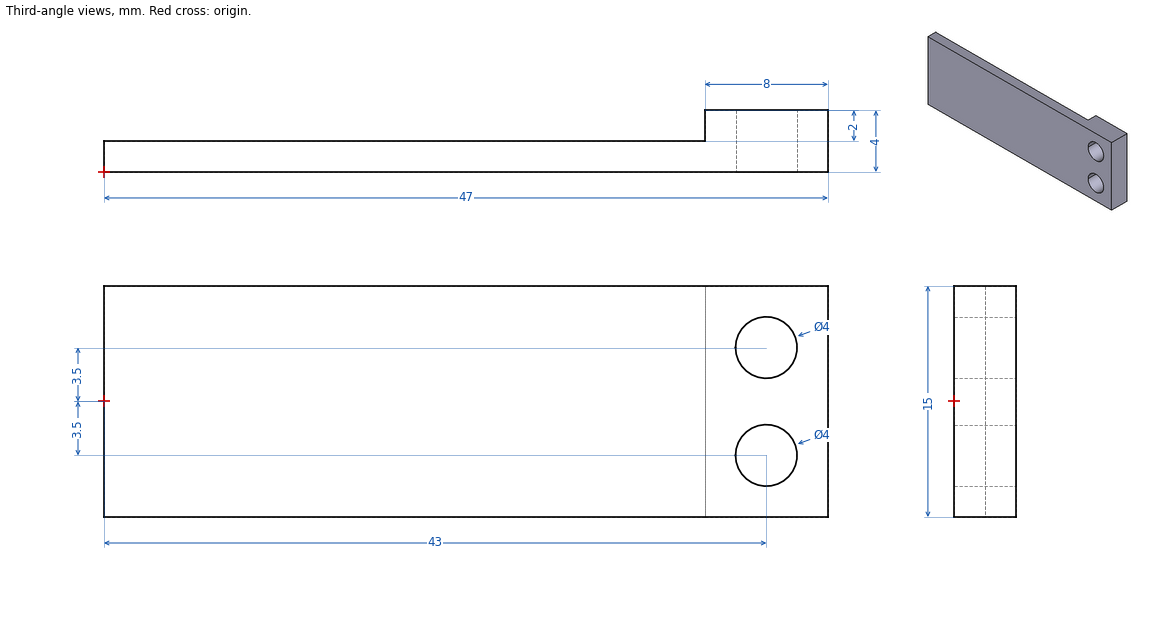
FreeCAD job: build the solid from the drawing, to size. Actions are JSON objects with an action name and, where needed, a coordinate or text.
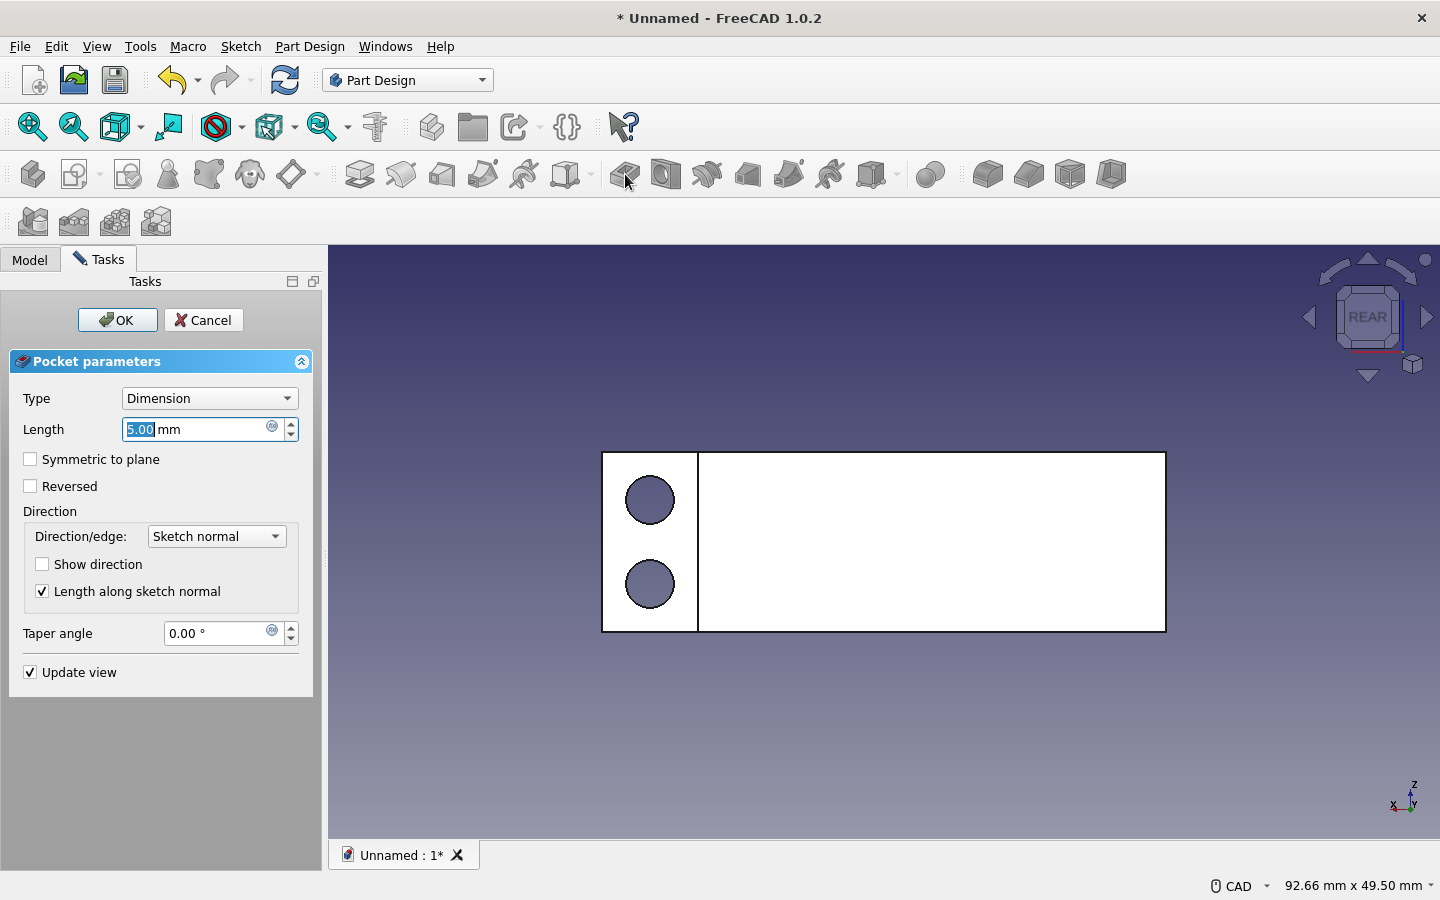
{"action": "left_click", "coordinate": [210, 398]}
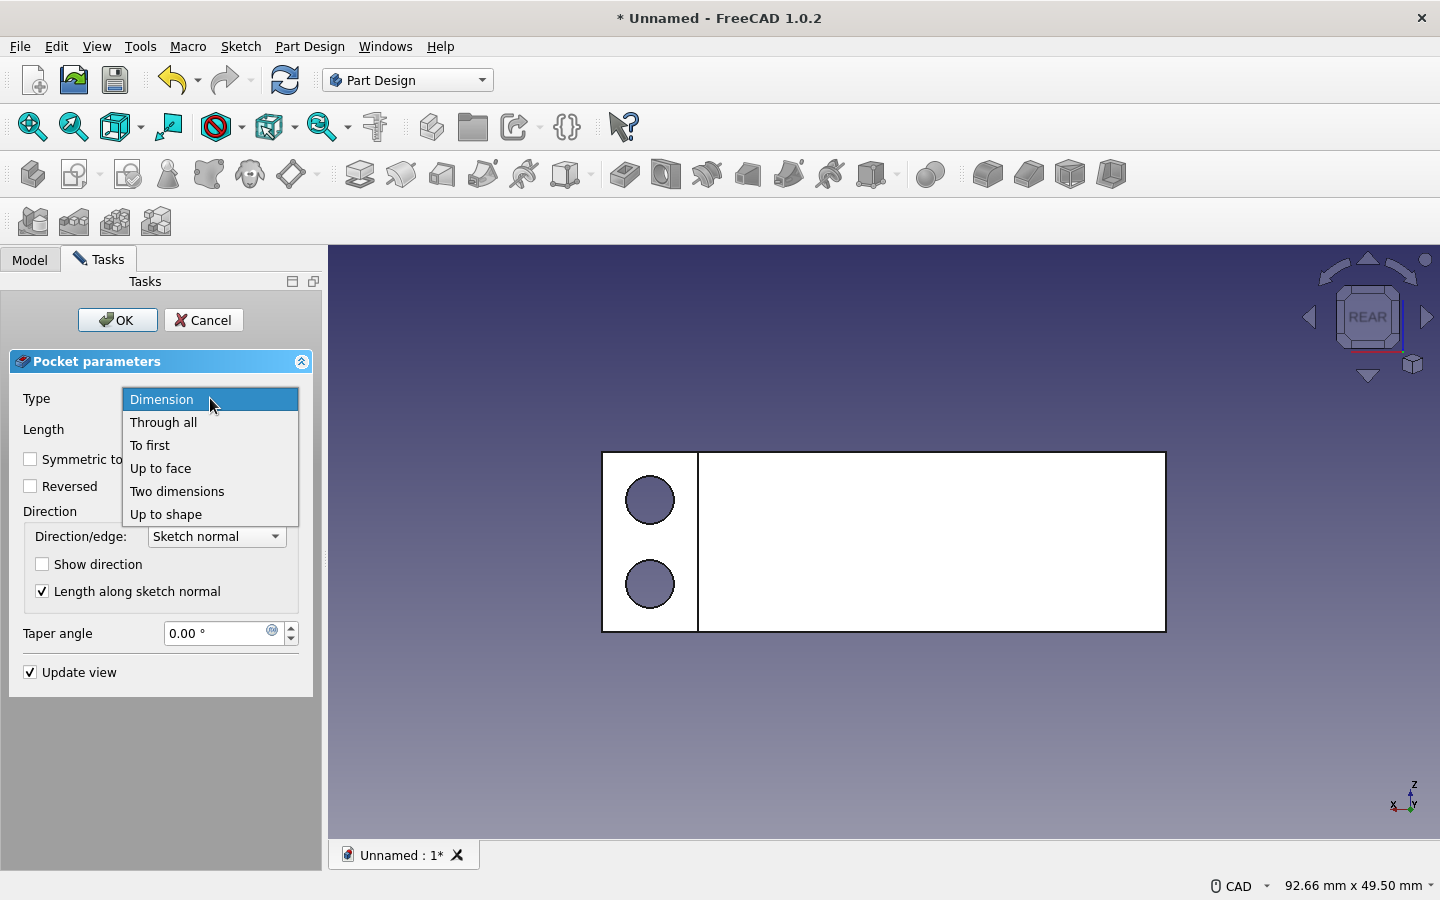
{"action": "left_click", "coordinate": [208, 446]}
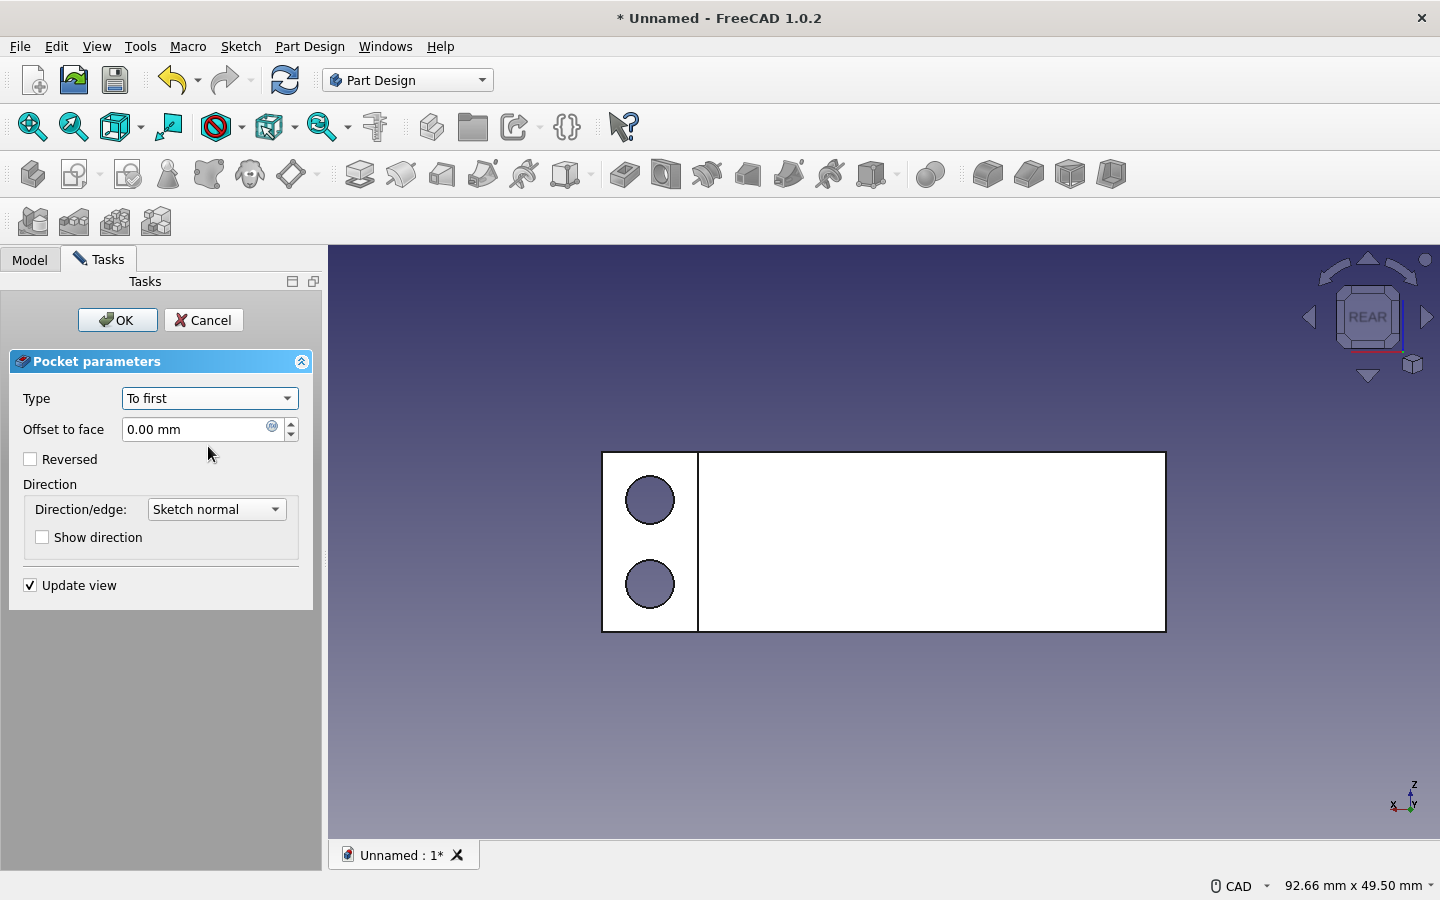
{"action": "left_click", "coordinate": [118, 320]}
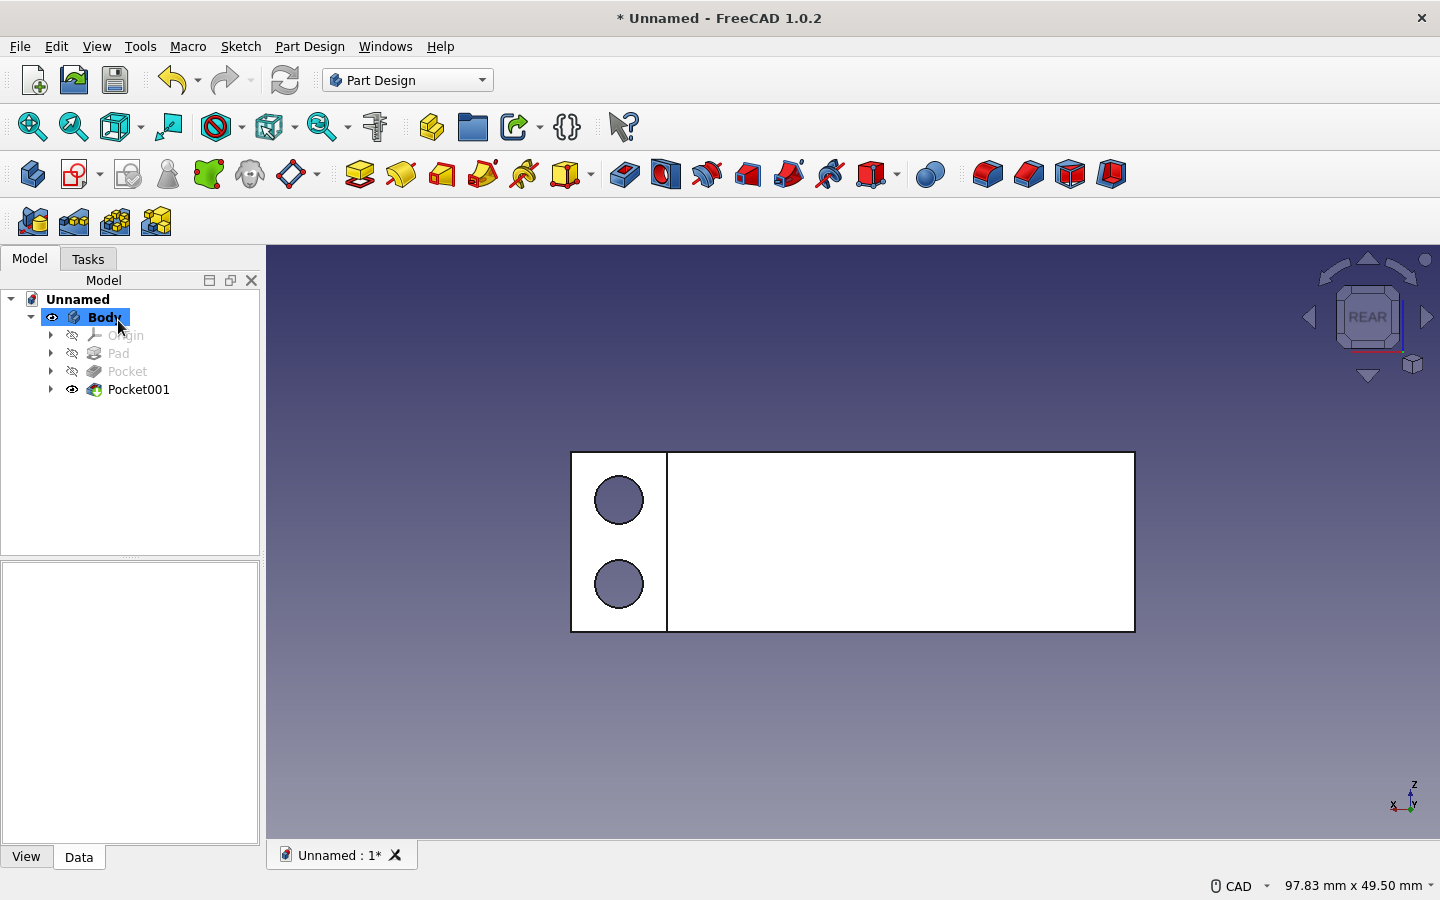
{"action": "key", "text": "0"}